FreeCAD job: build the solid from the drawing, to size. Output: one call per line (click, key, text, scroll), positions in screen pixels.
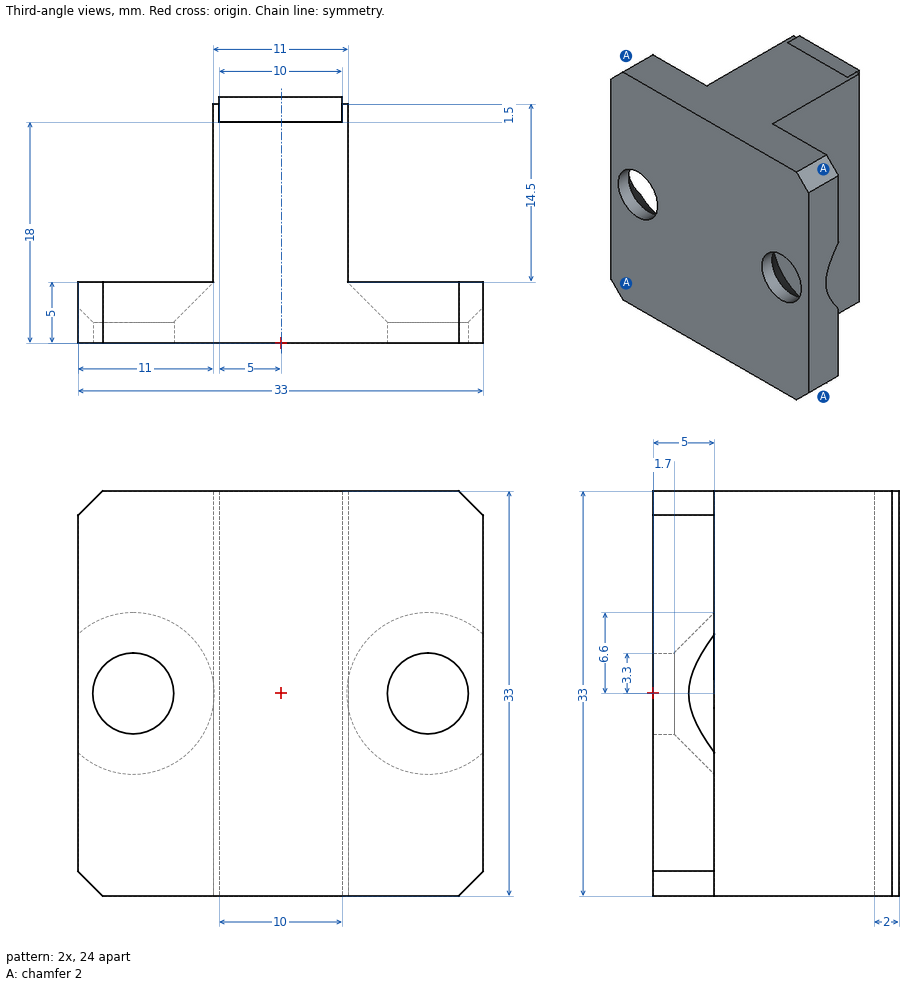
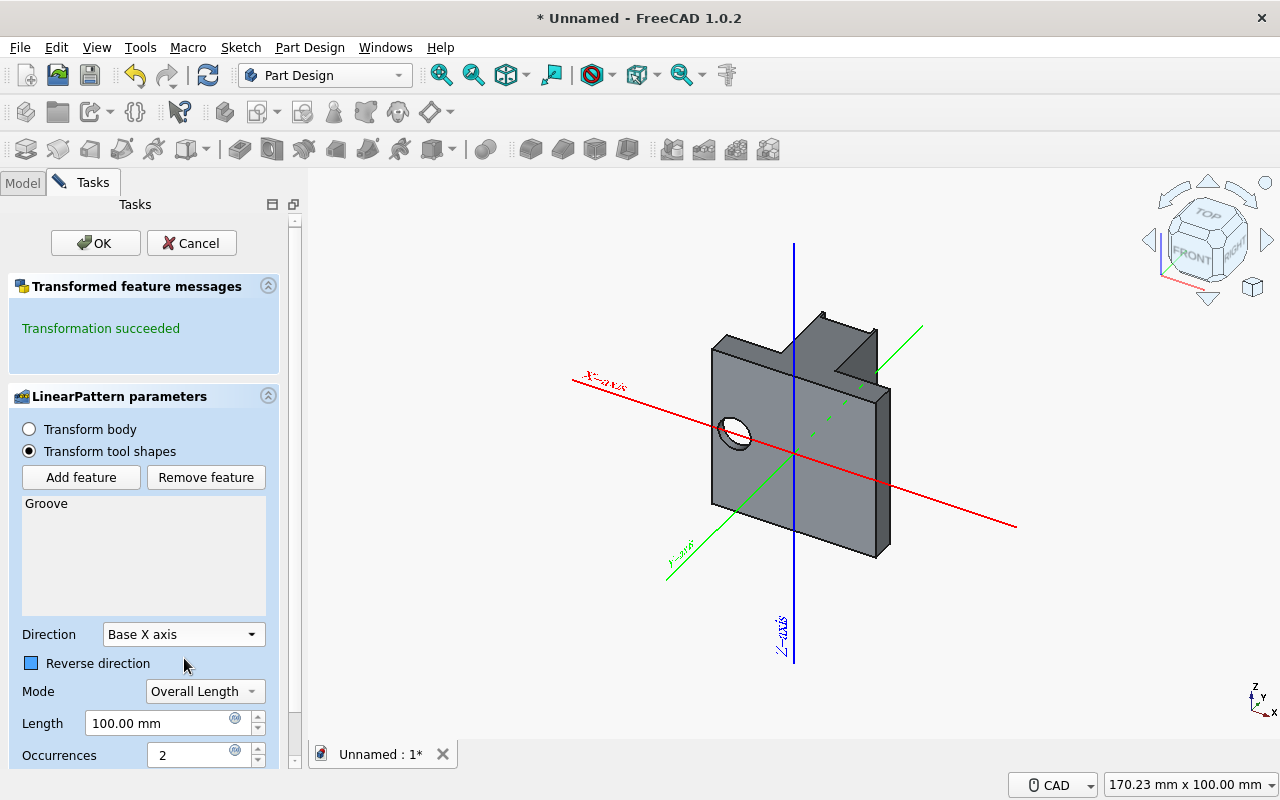
click(206, 692)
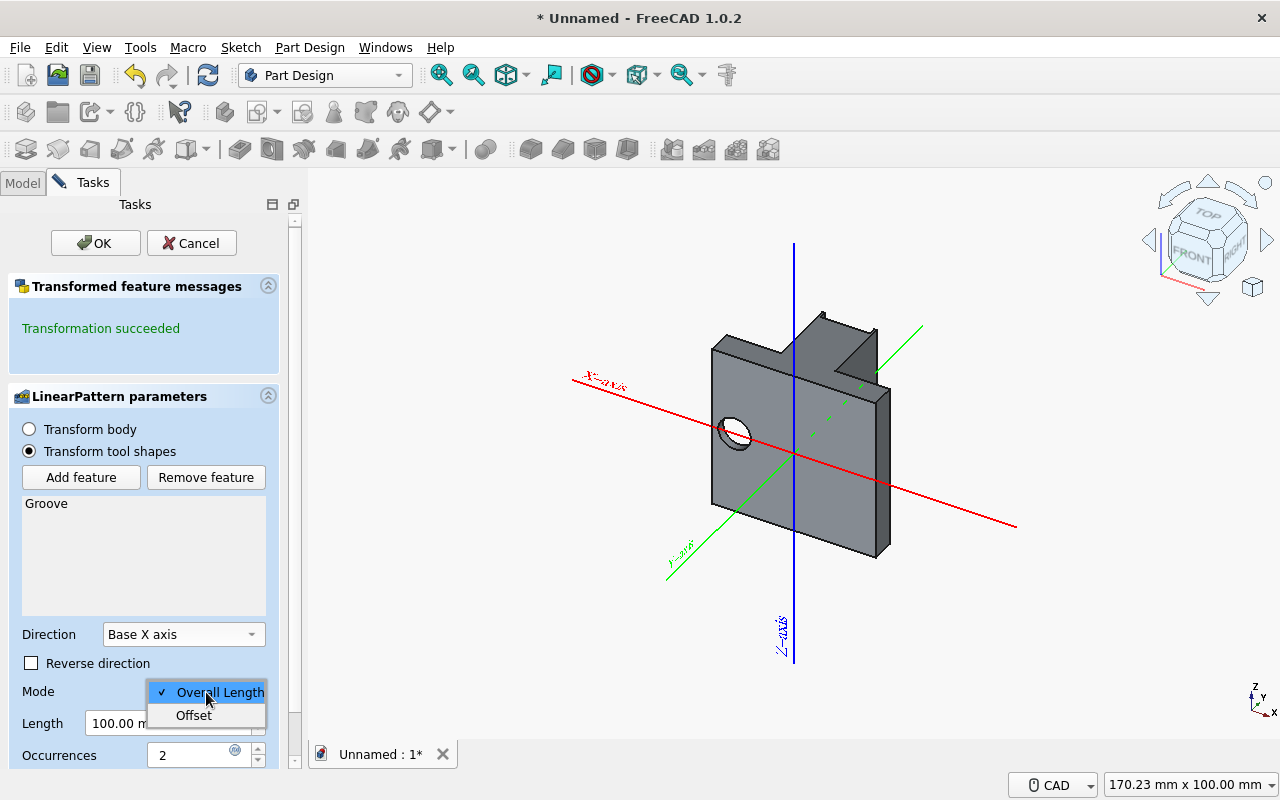
click(206, 716)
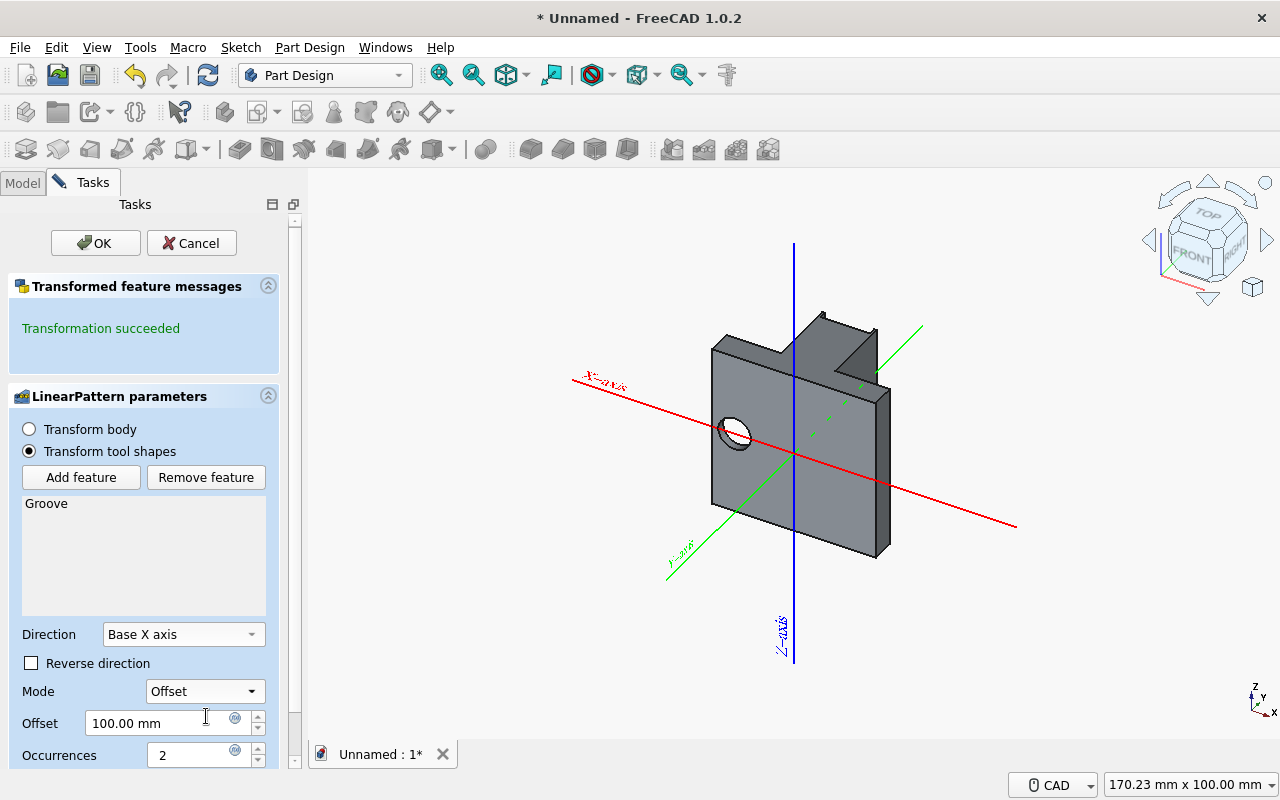
triple_click(168, 723)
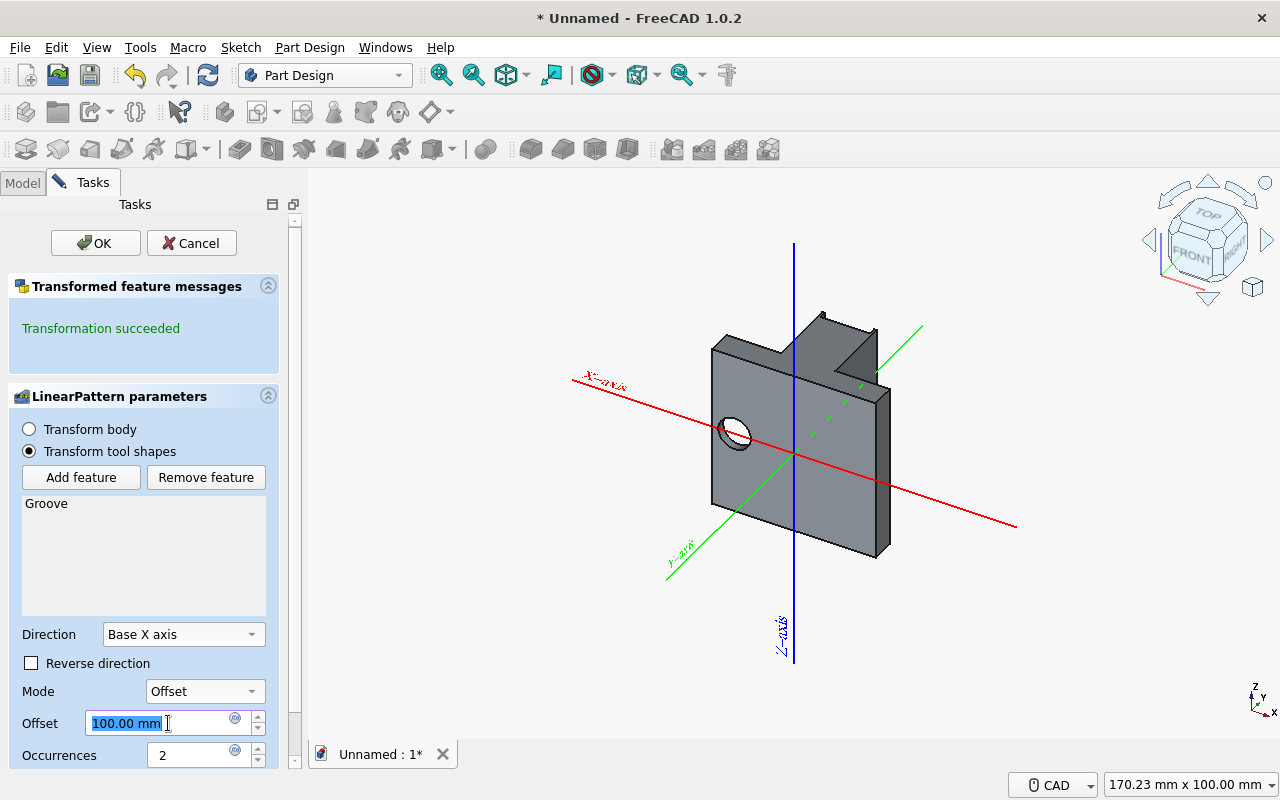
text(24)
key(Tab)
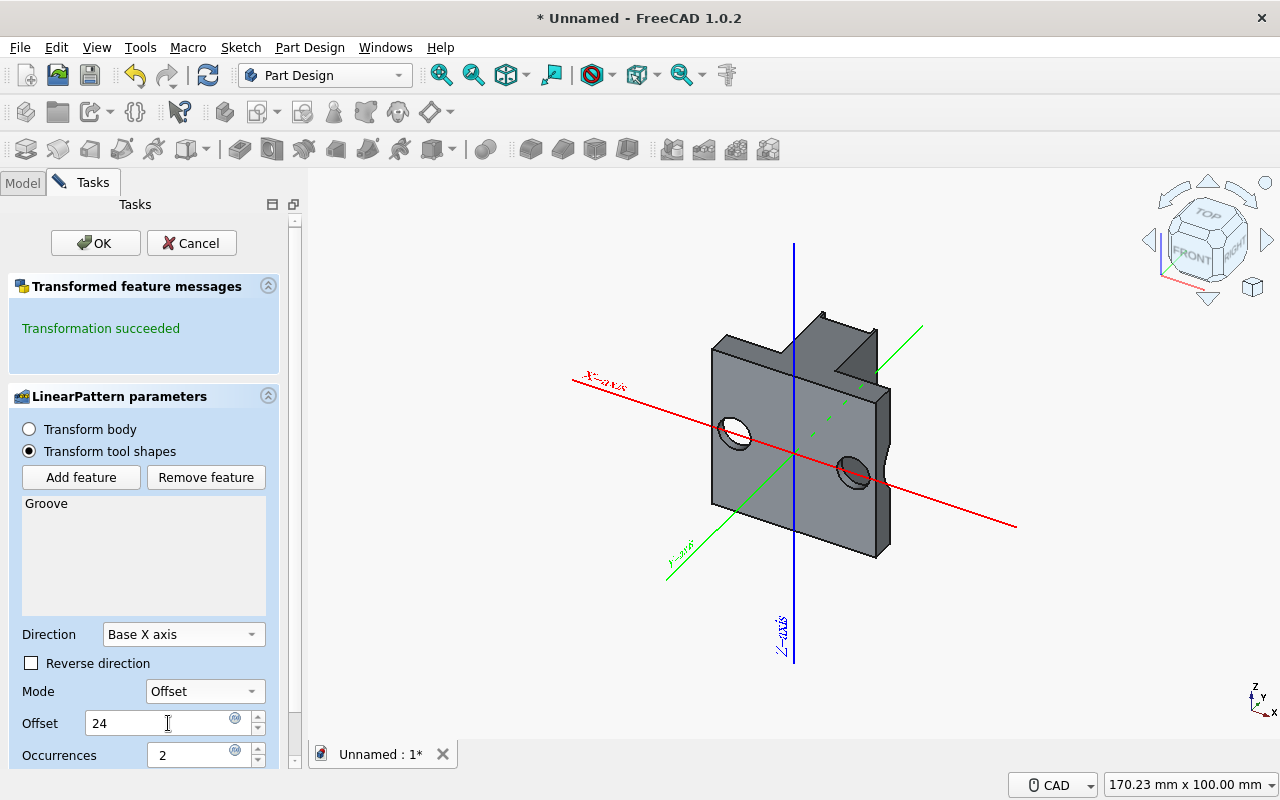
triple_click(198, 755)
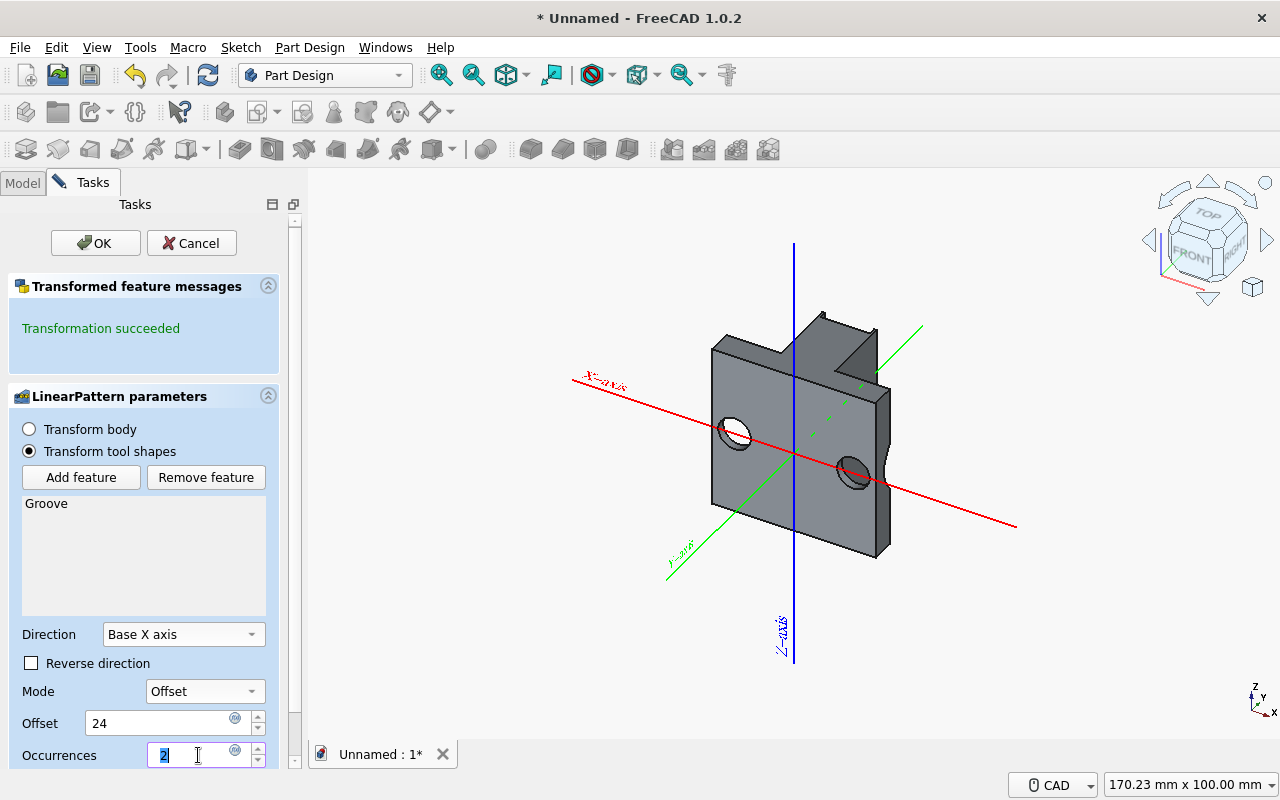
text(2)
key(Tab)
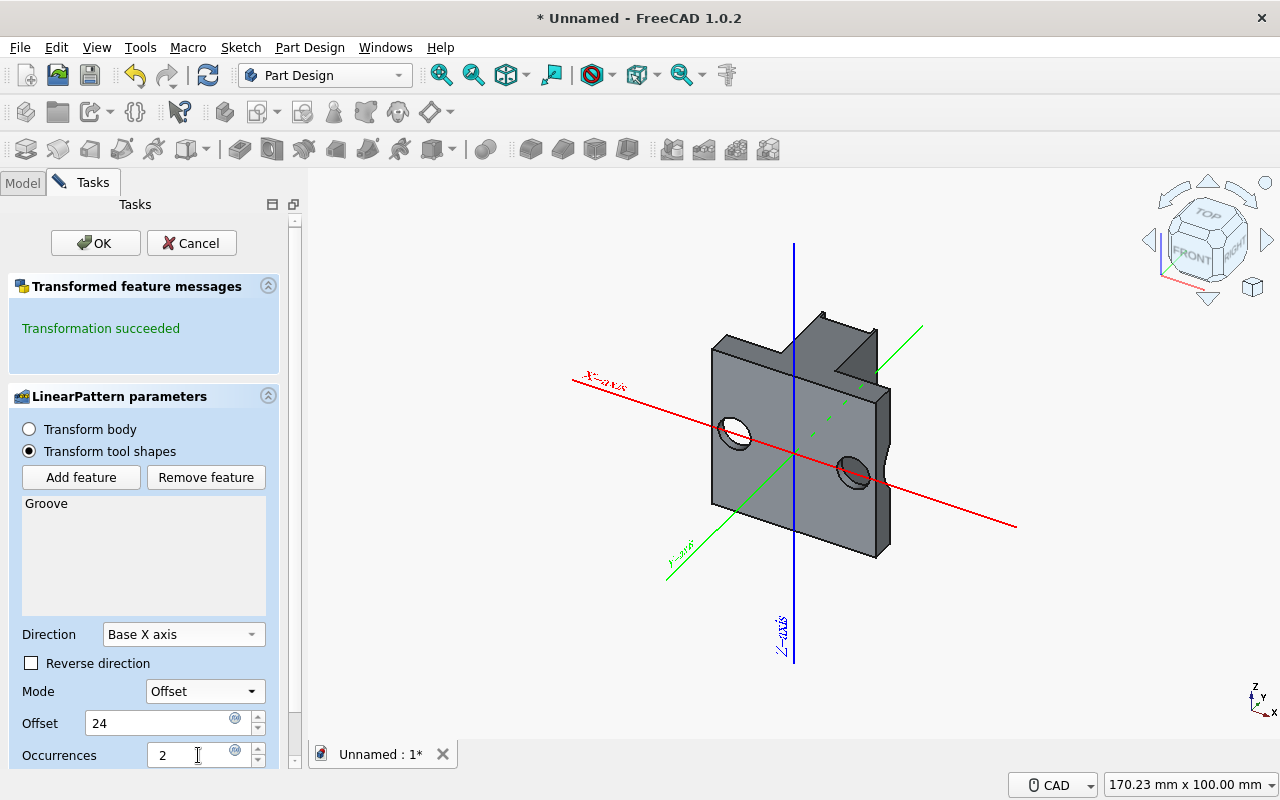
click(96, 243)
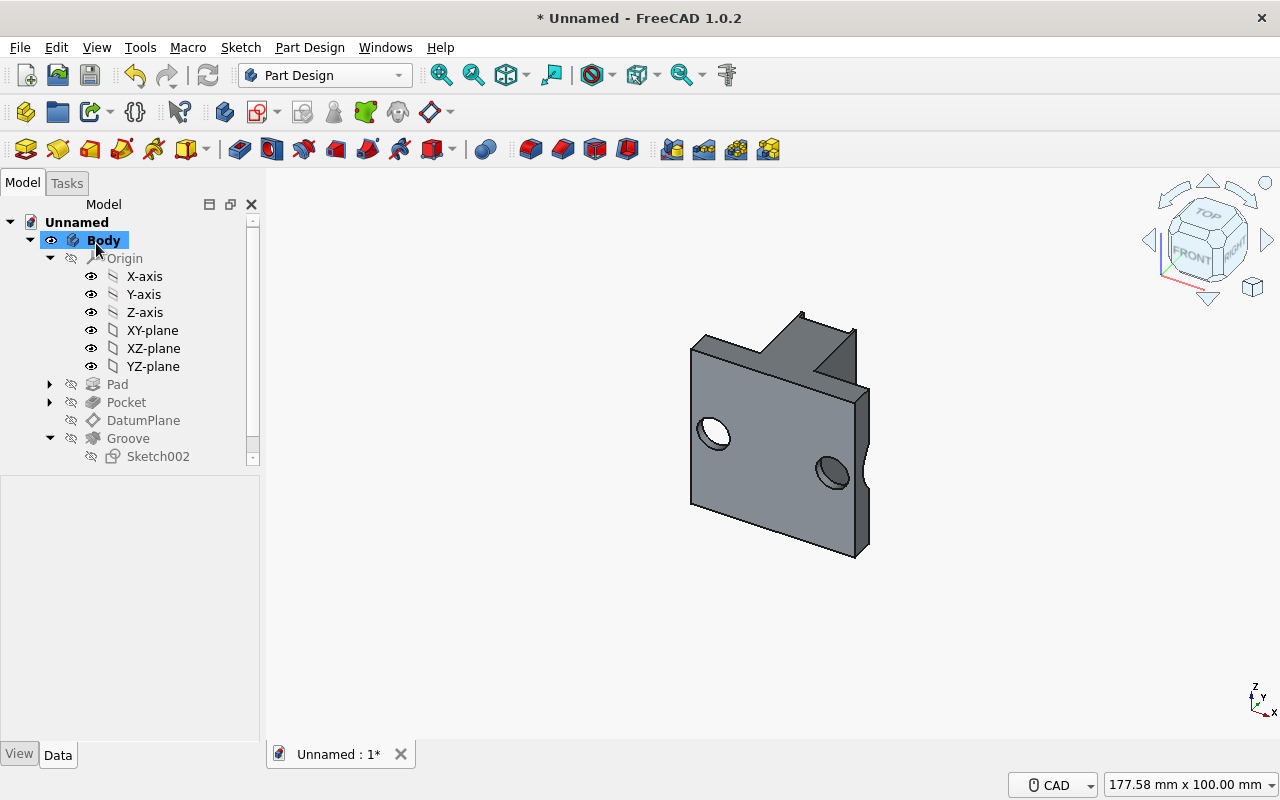
click(862, 395)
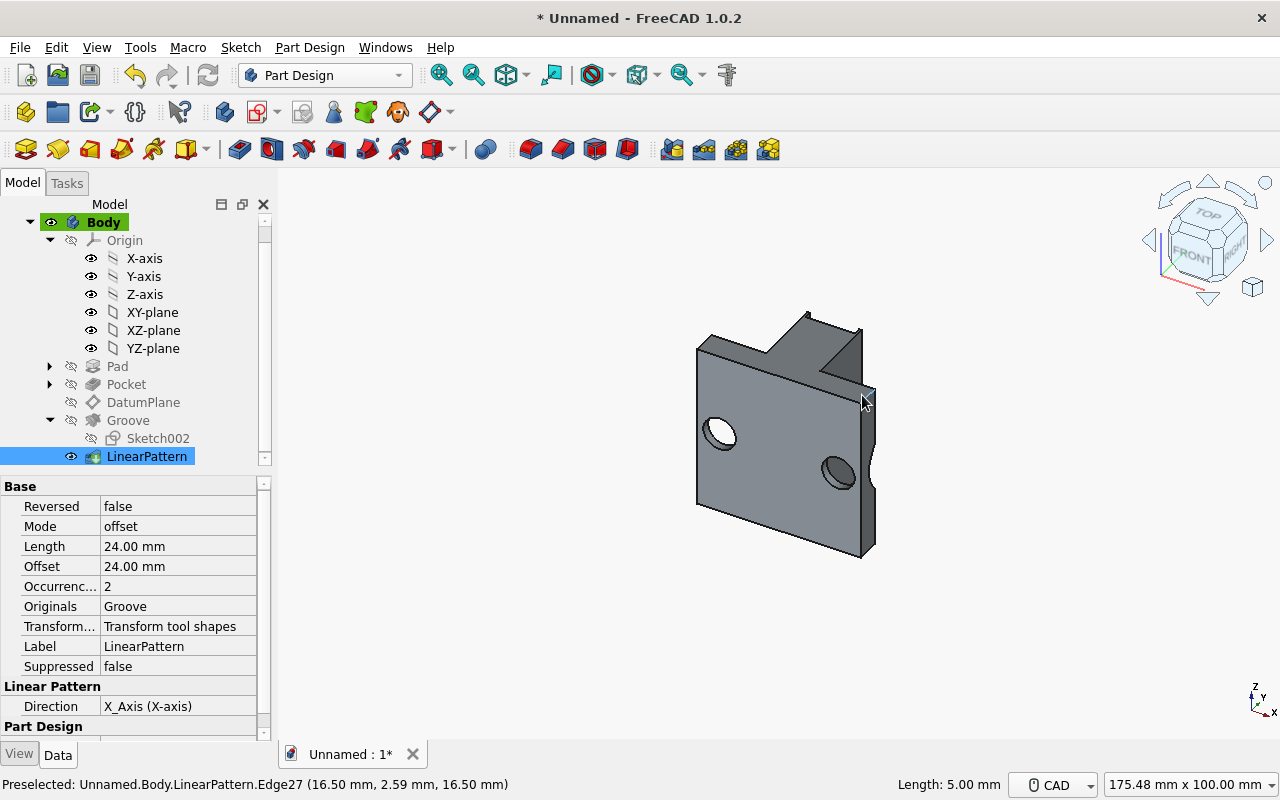
key(0)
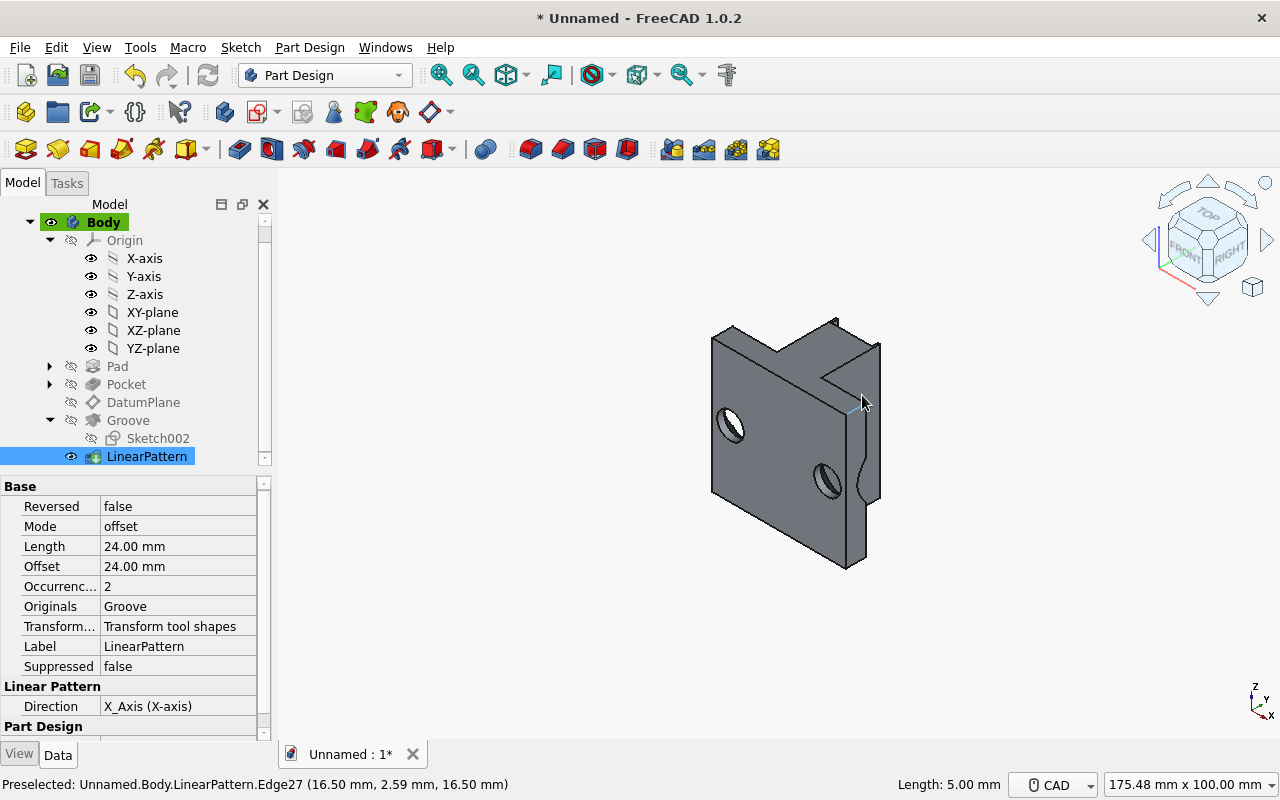
key(2)